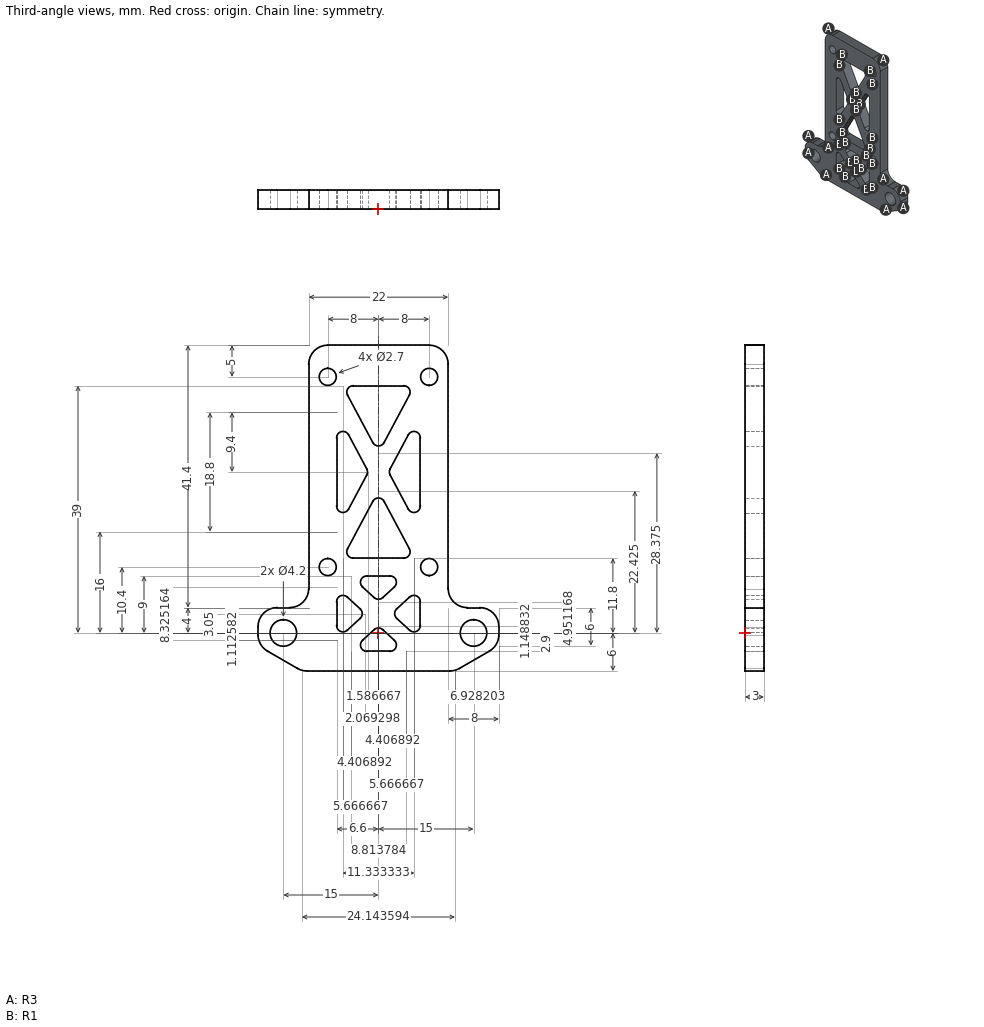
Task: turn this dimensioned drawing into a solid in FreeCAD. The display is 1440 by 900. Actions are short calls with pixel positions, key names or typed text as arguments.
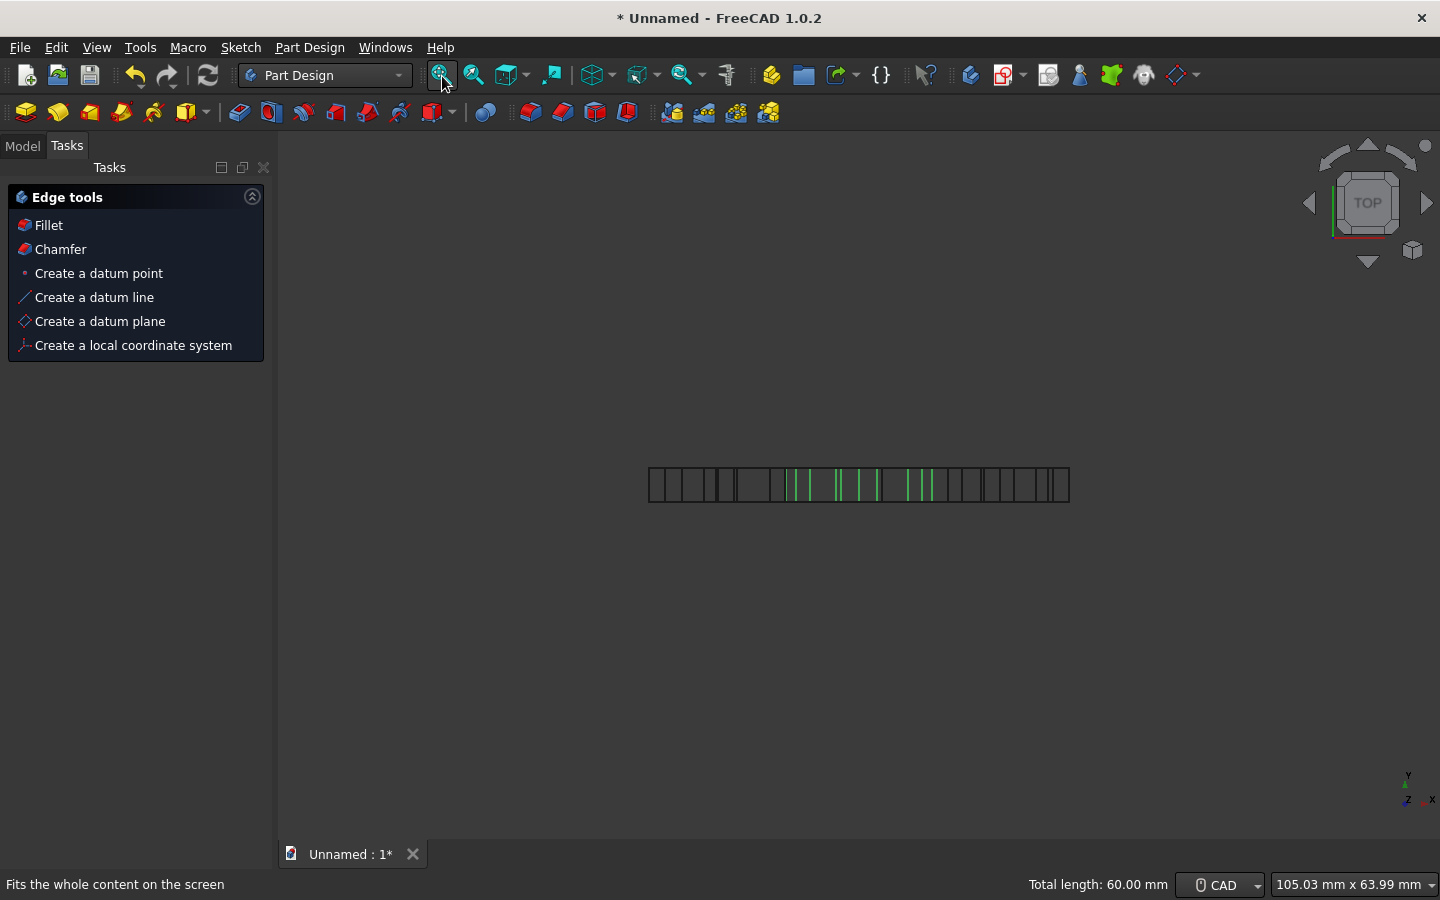
scroll(786, 484, up, 6)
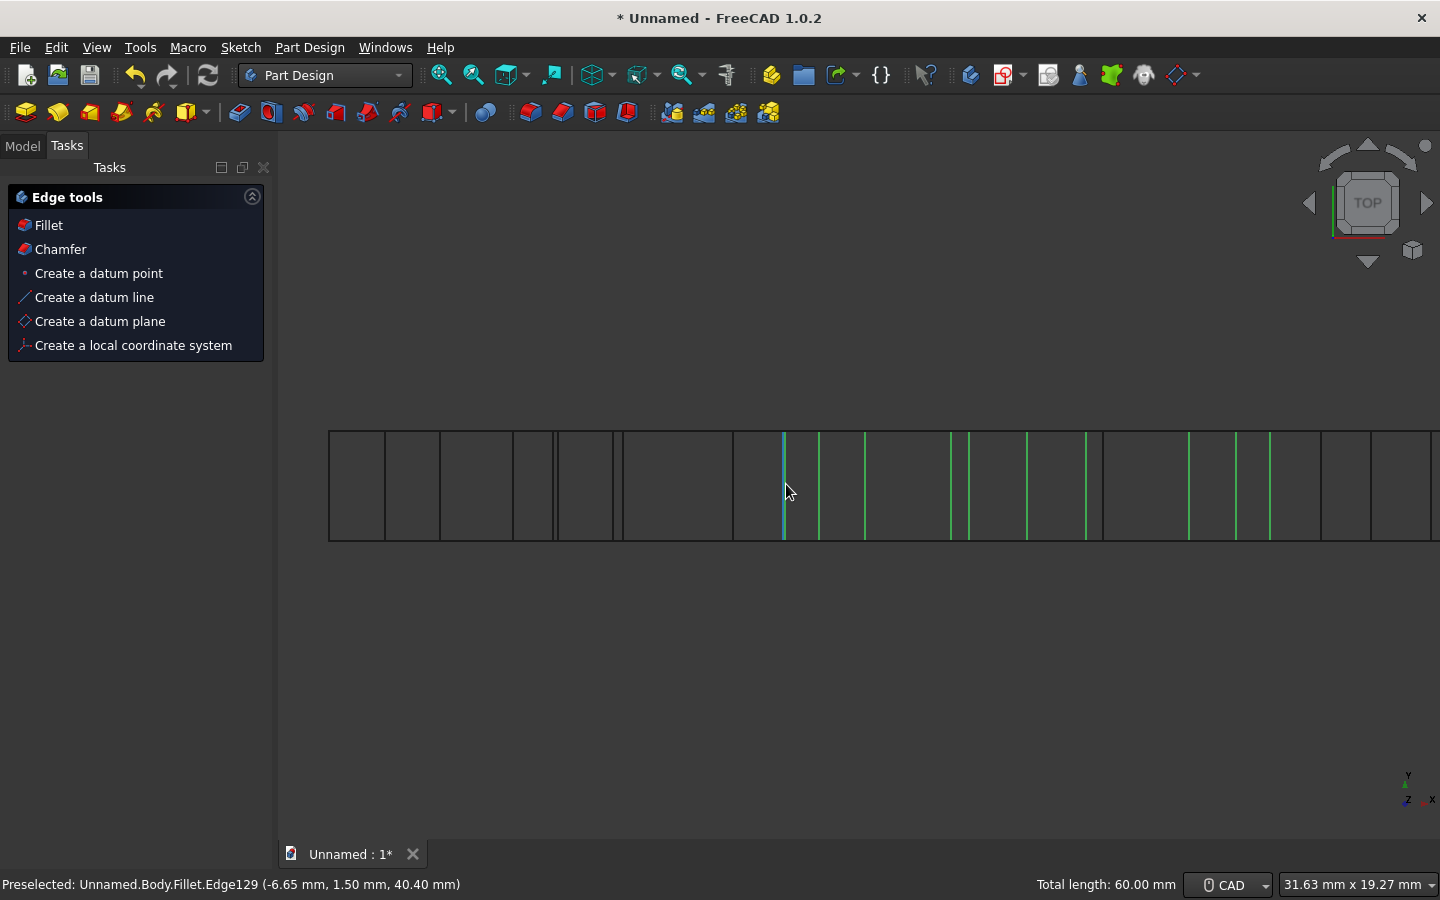
click(1103, 485, ctrl)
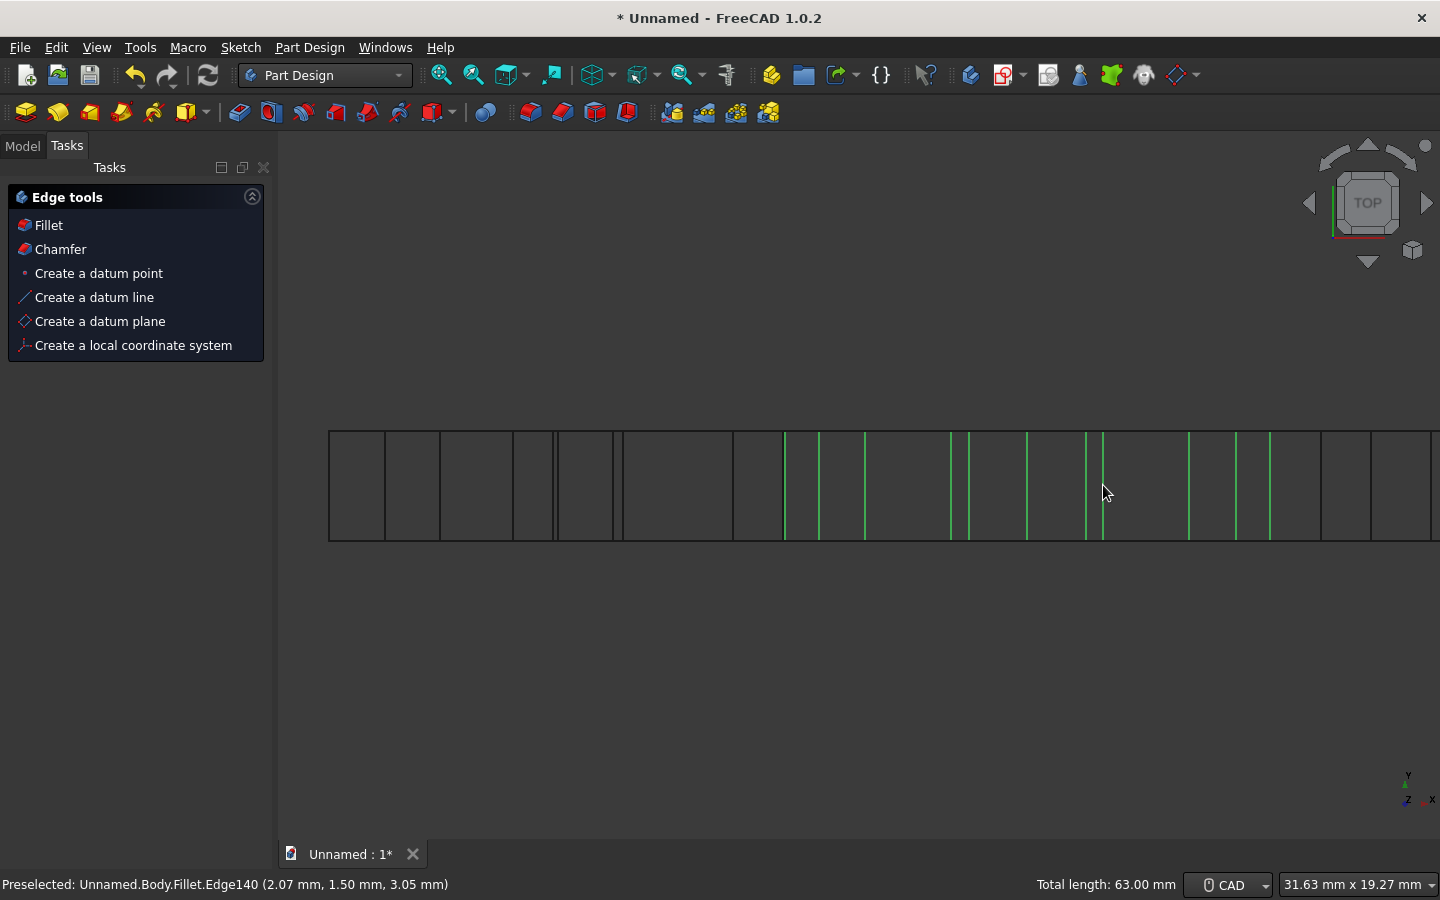
click(442, 76)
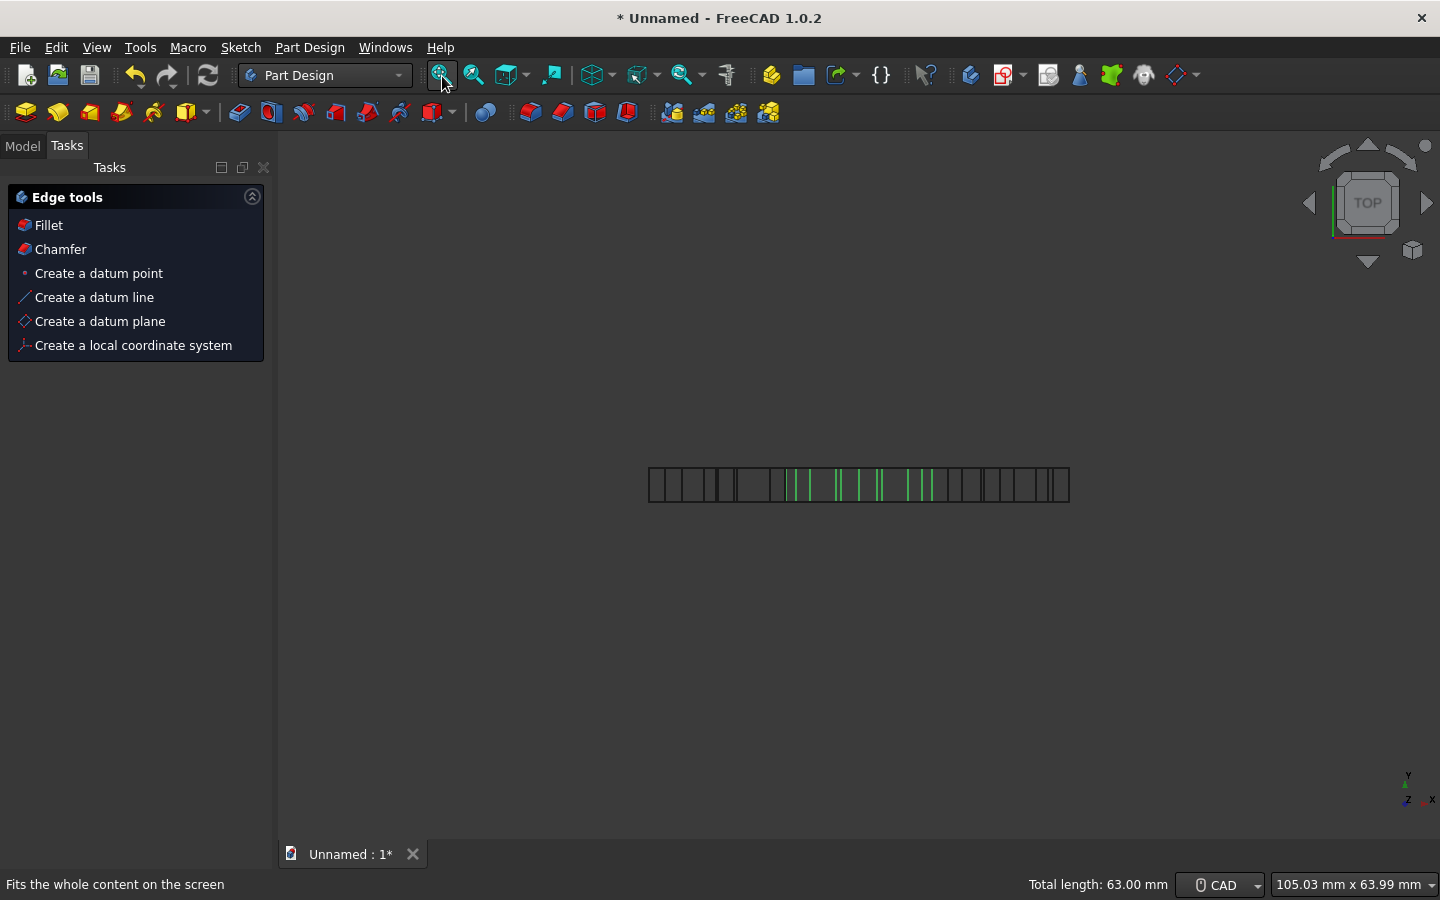
key(1)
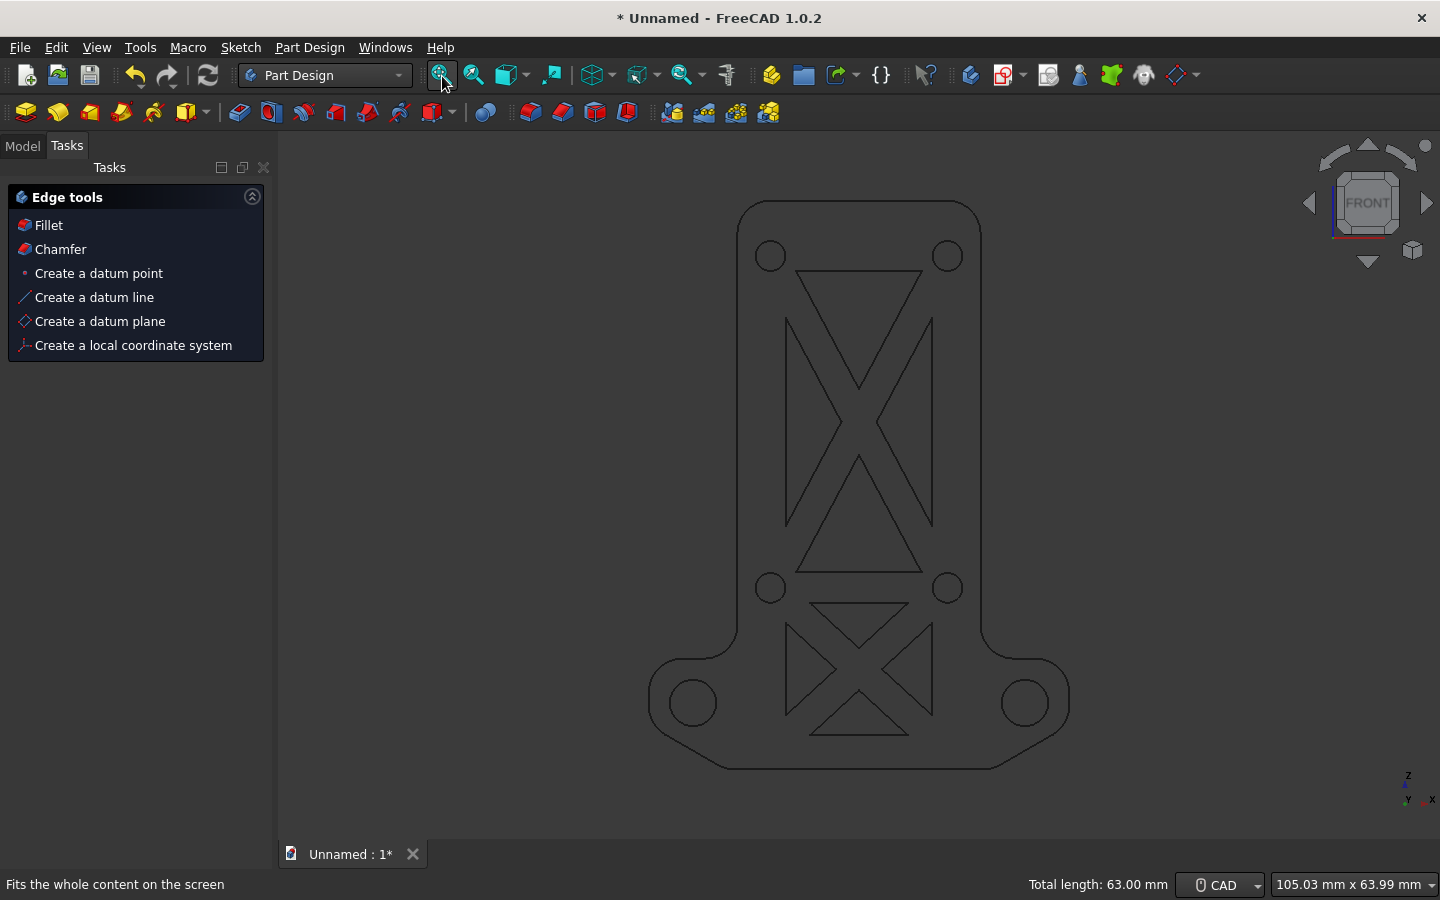
scroll(786, 714, up, 6)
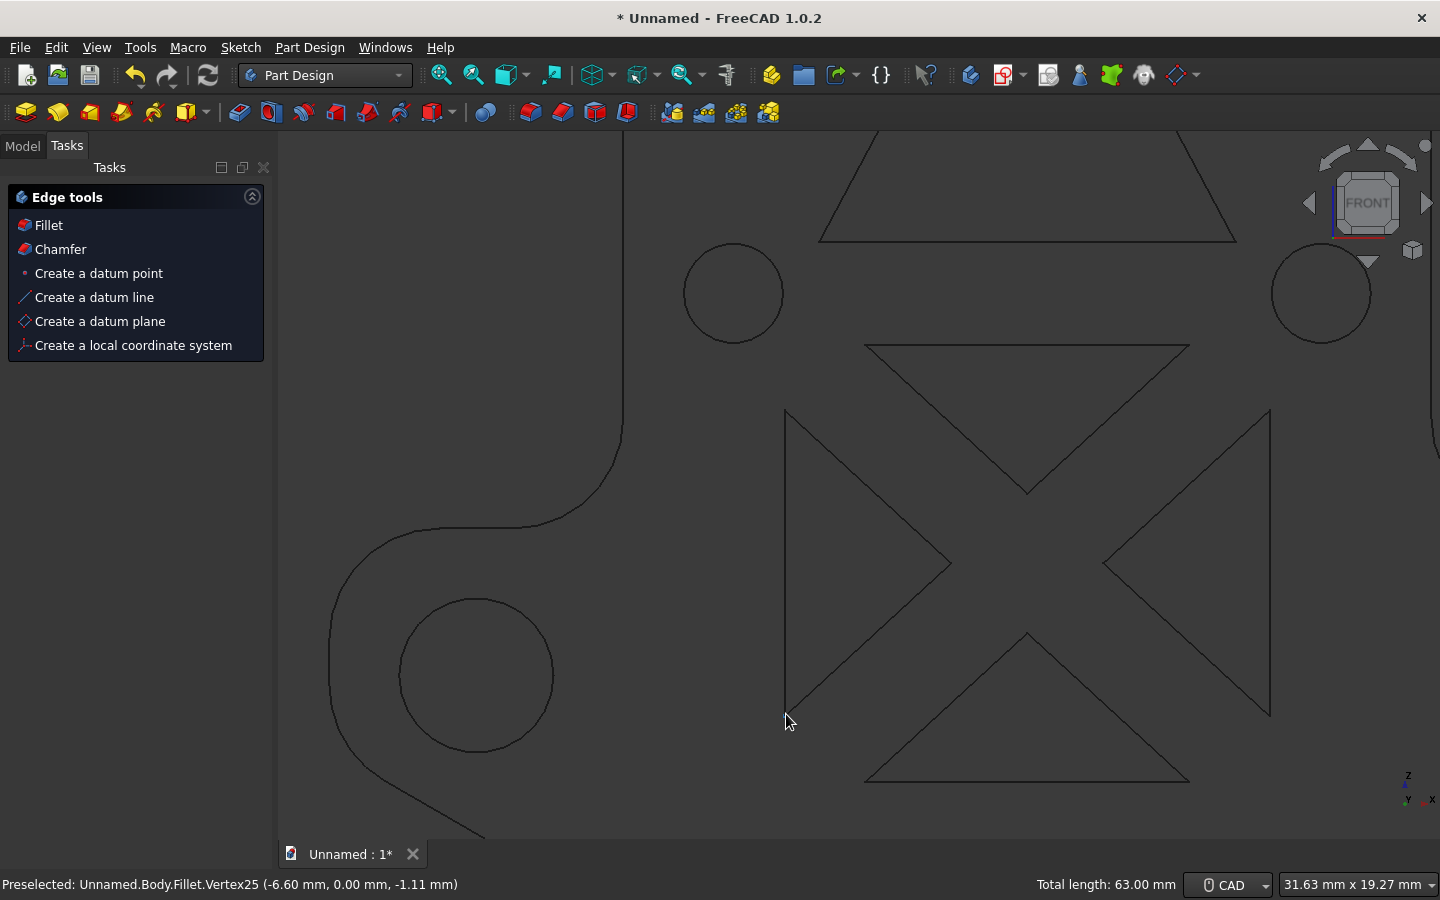
click(442, 76)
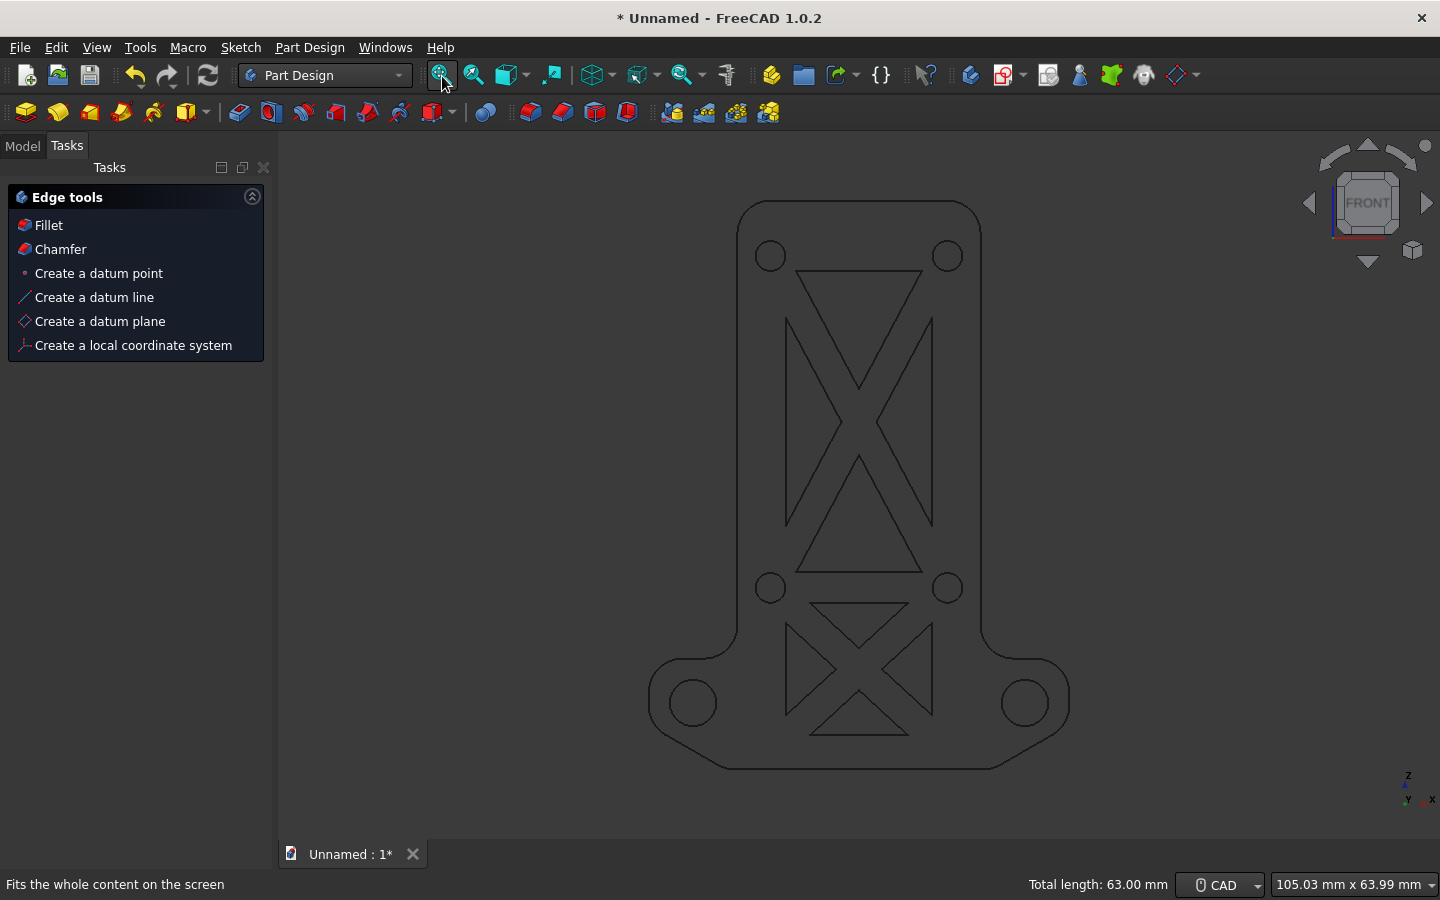
key(3)